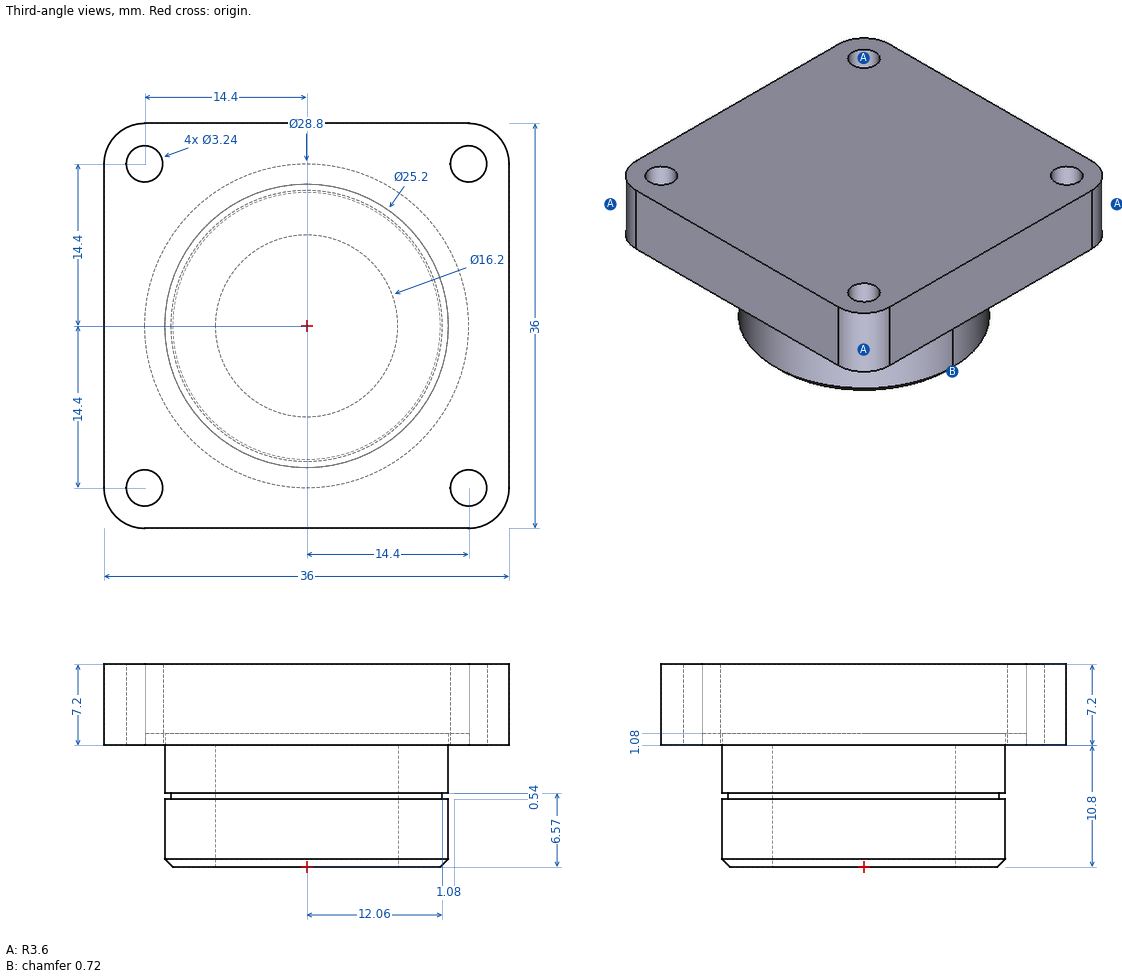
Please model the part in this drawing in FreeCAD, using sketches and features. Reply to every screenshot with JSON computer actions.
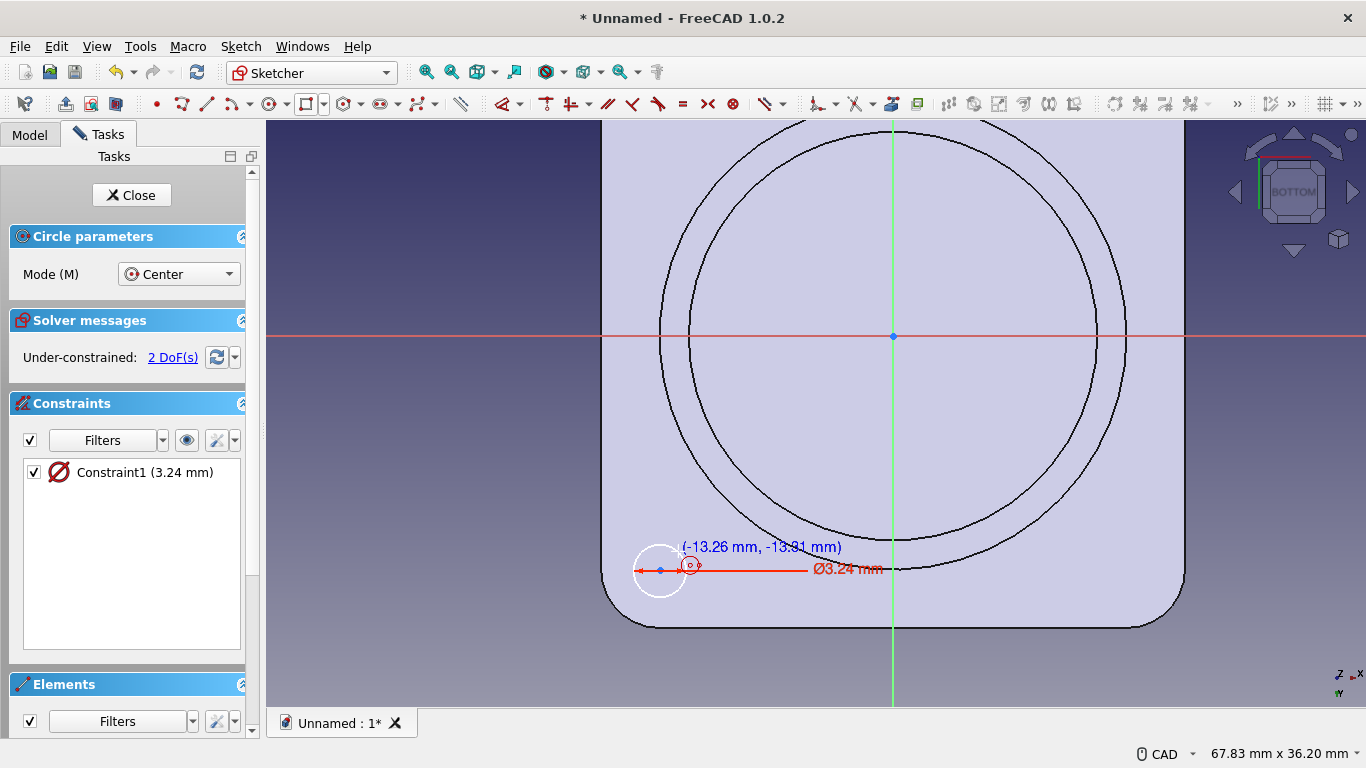
{"action": "scroll", "coordinate": [452, 571], "scroll_direction": "down", "scroll_amount": 2}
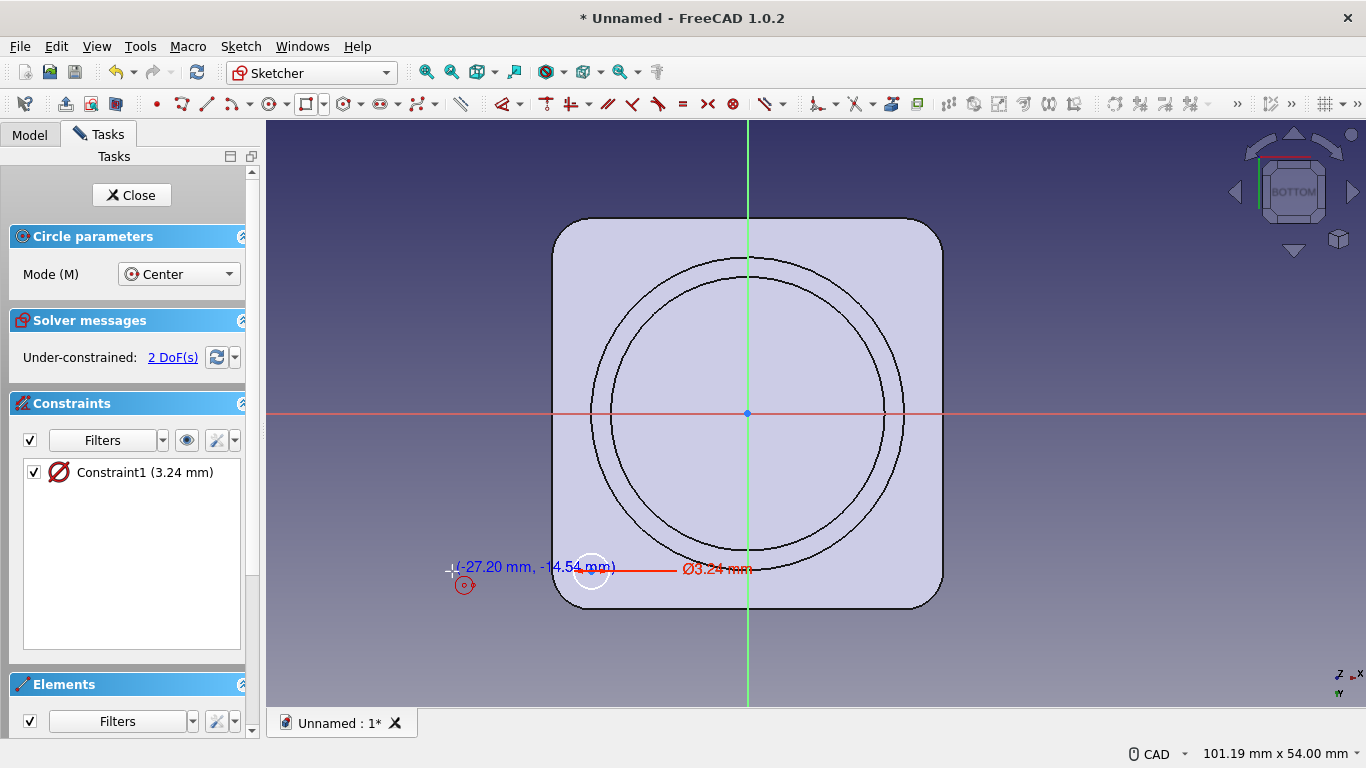
{"action": "scroll", "coordinate": [591, 257], "scroll_direction": "up", "scroll_amount": 2}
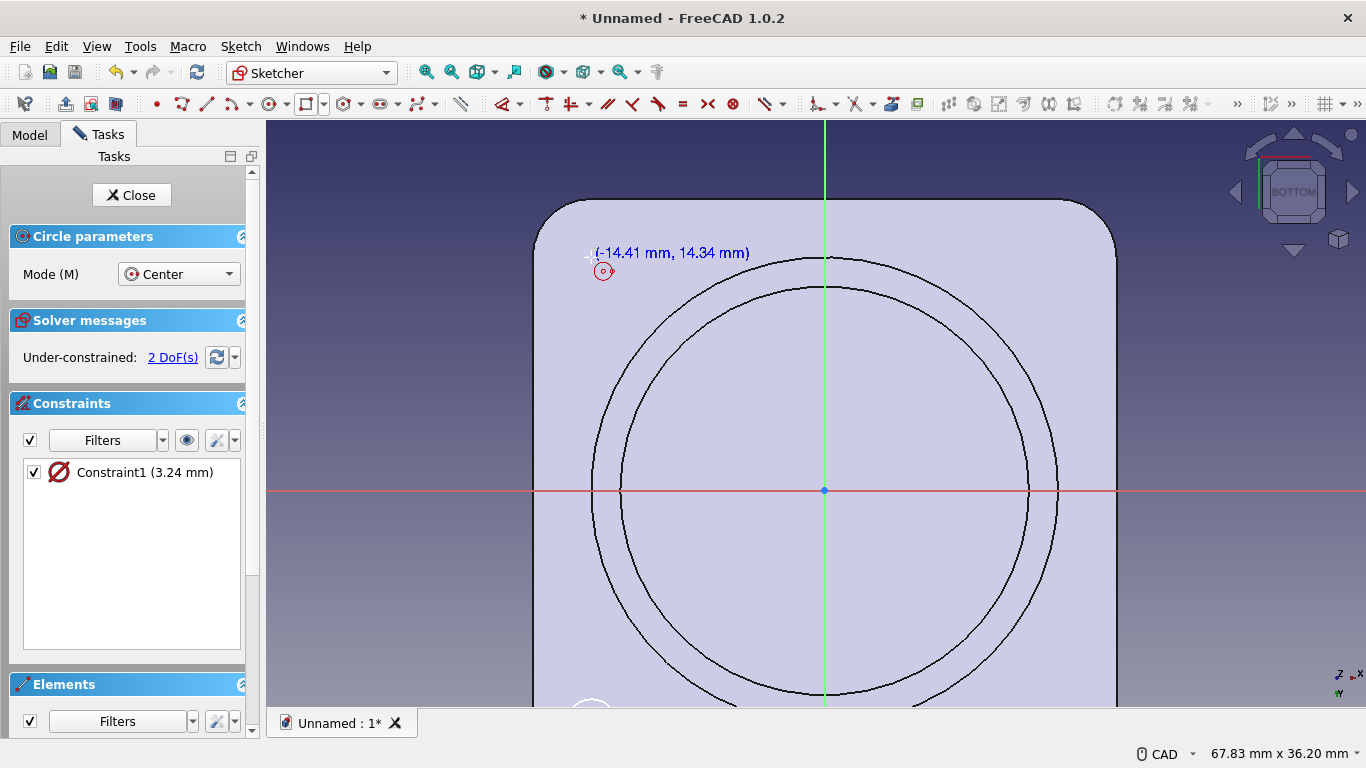
{"action": "left_click", "coordinate": [591, 257]}
{"action": "mouse_move", "coordinate": [610, 239]}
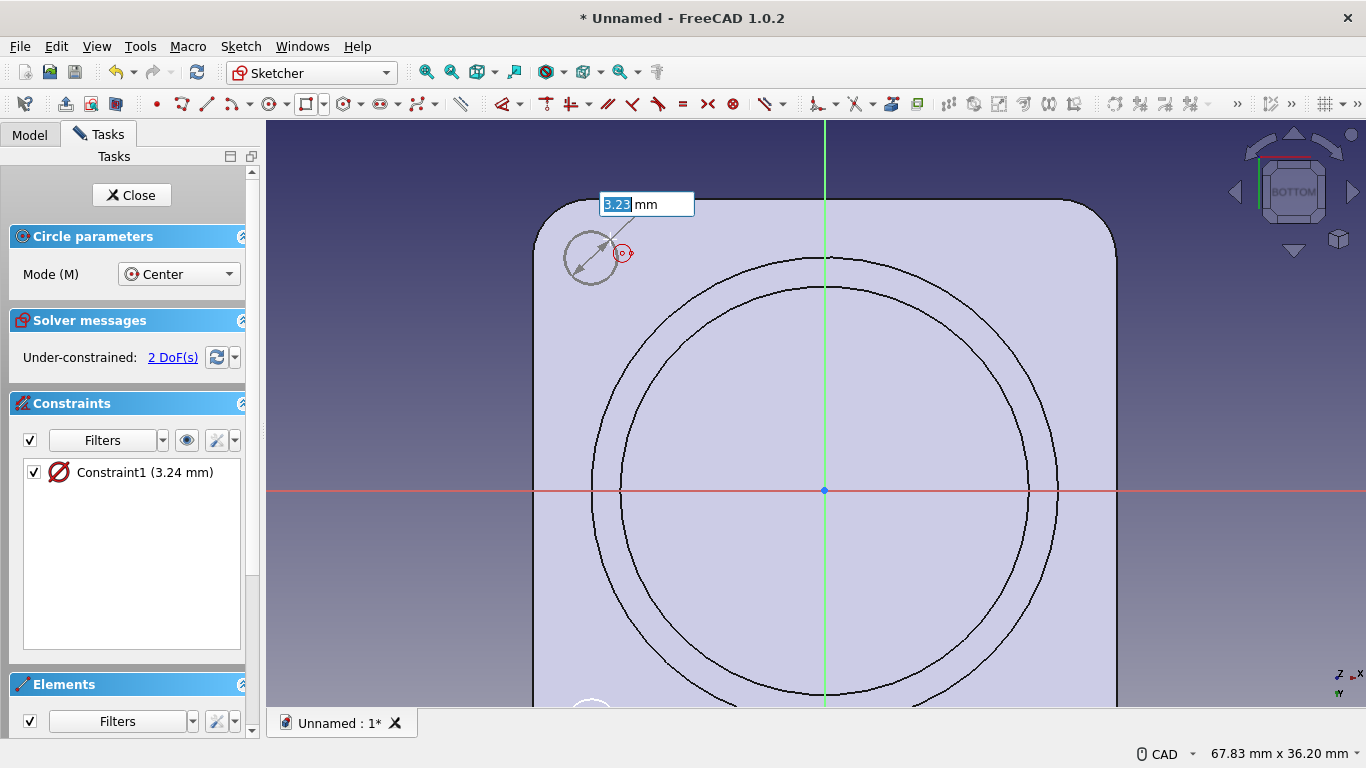
{"action": "type", "text": "3.24"}
{"action": "key", "text": "Return"}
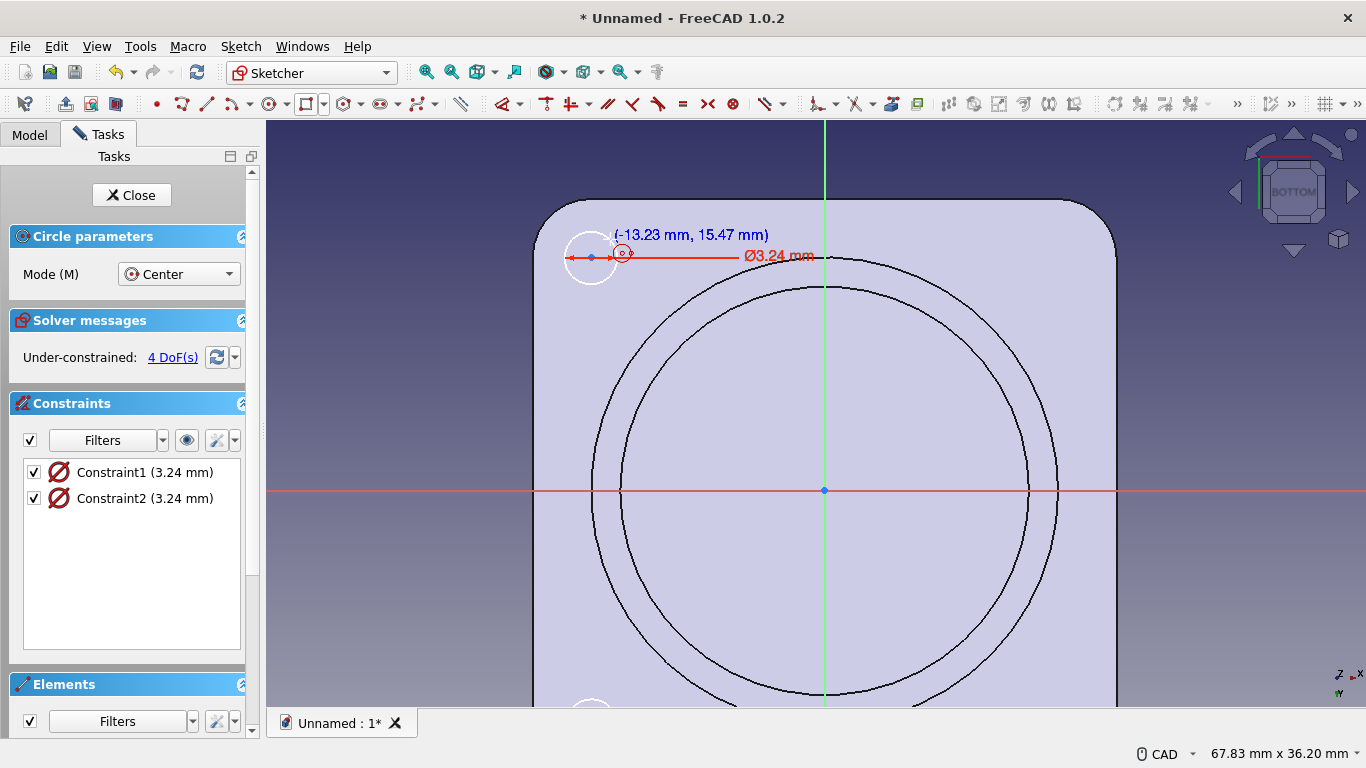
{"action": "left_click", "coordinate": [1058, 257]}
{"action": "mouse_move", "coordinate": [1077, 239]}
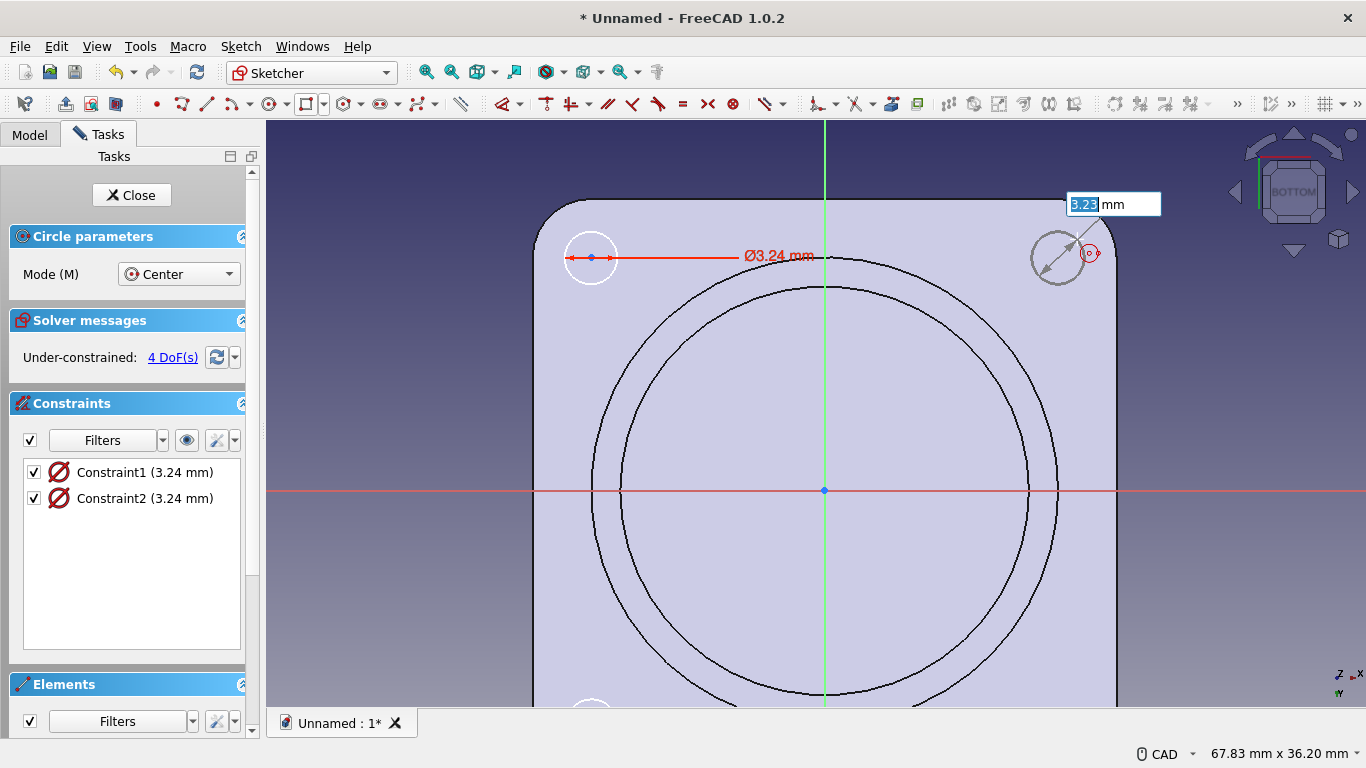
{"action": "type", "text": "3.24"}
{"action": "key", "text": "Return"}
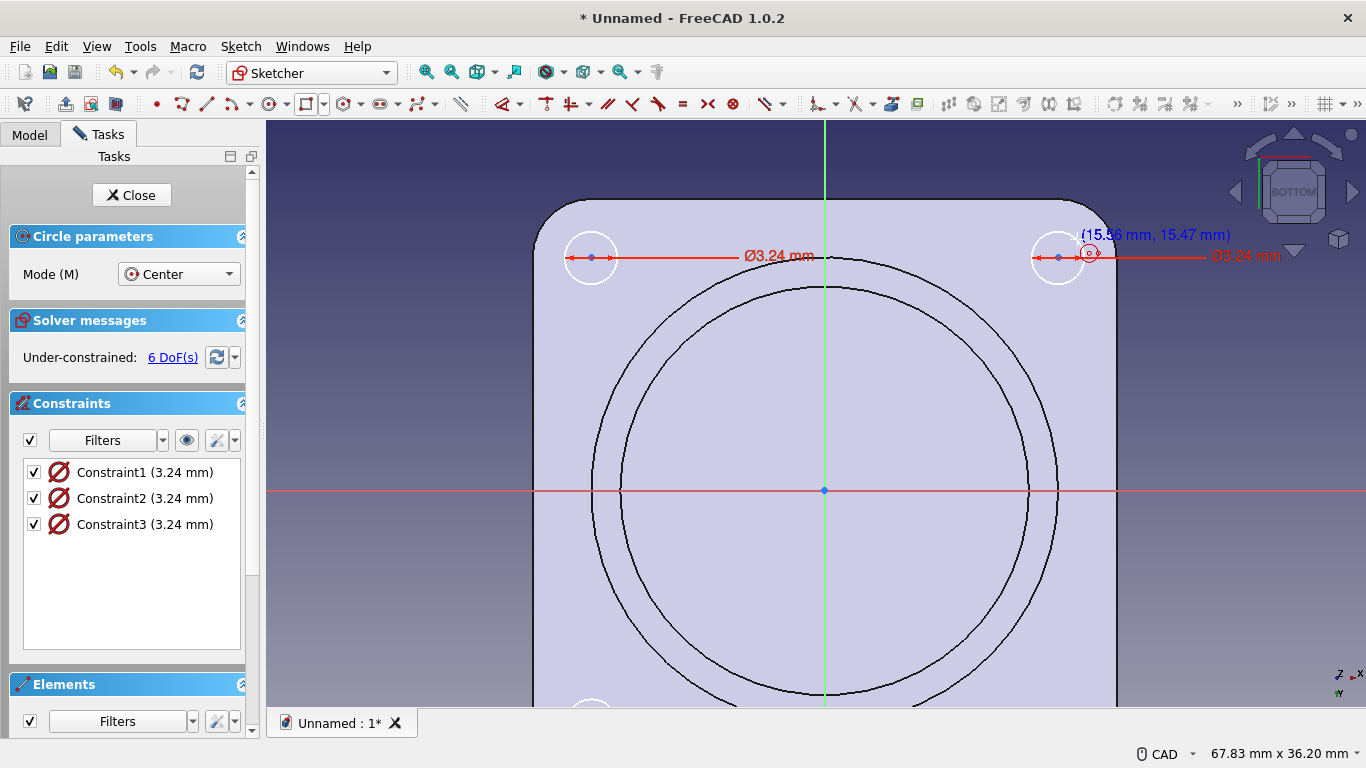
{"action": "scroll", "coordinate": [591, 256], "scroll_direction": "down", "scroll_amount": 2}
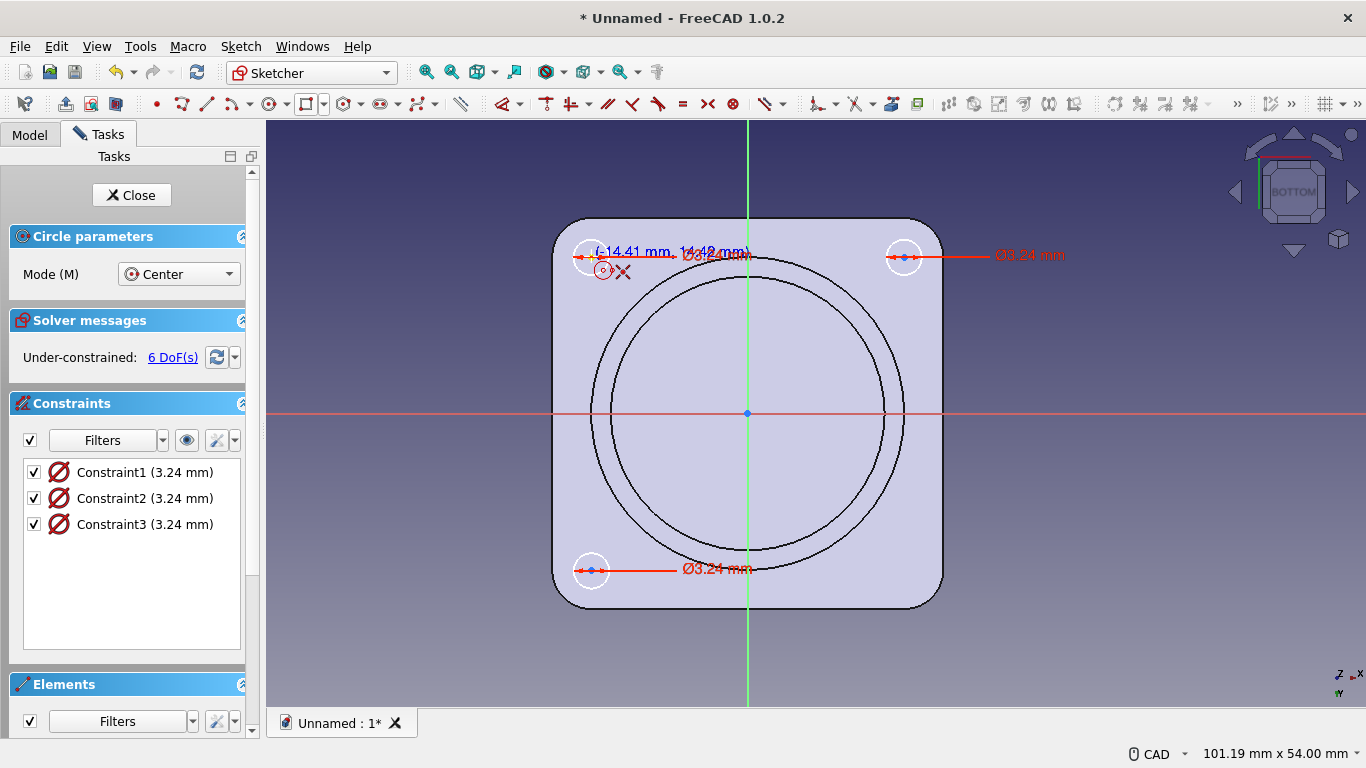
{"action": "scroll", "coordinate": [904, 570], "scroll_direction": "up", "scroll_amount": 2}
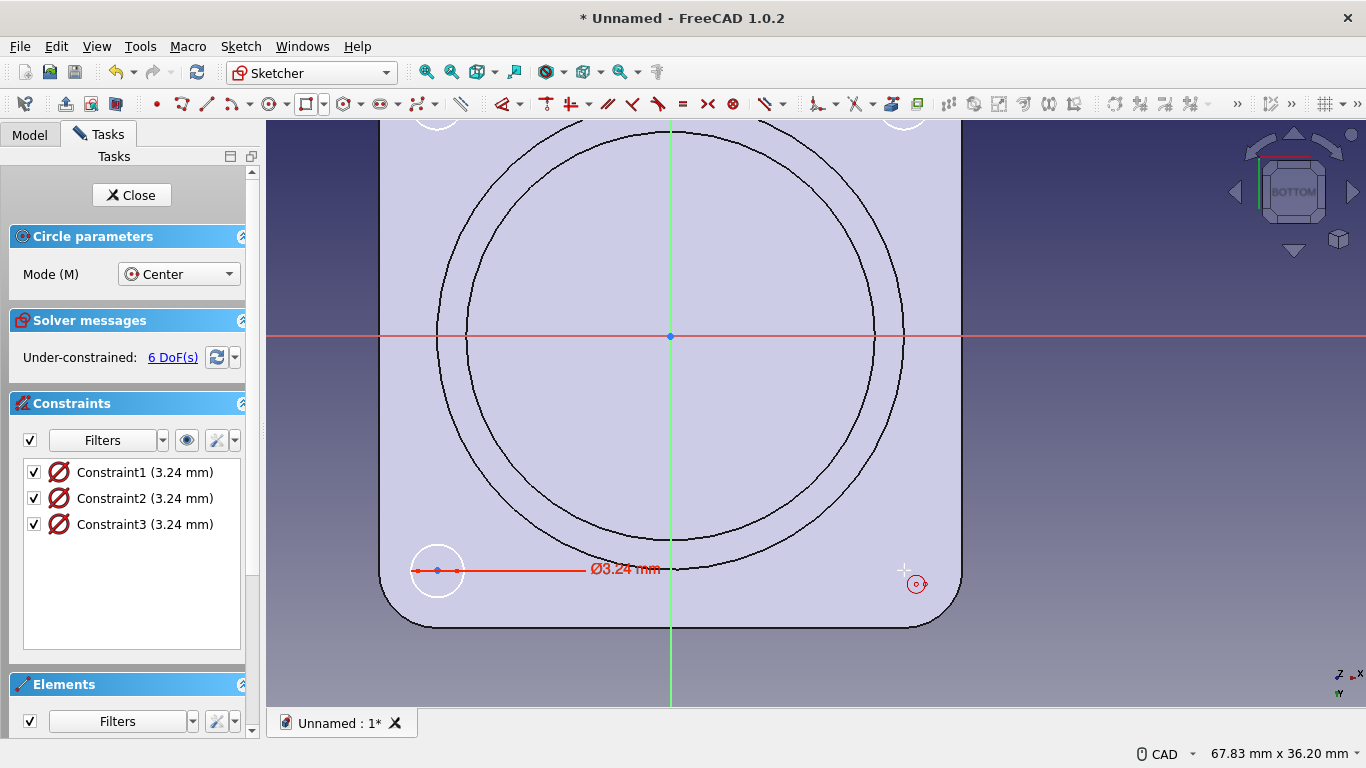
{"action": "left_click", "coordinate": [904, 570]}
{"action": "mouse_move", "coordinate": [923, 551]}